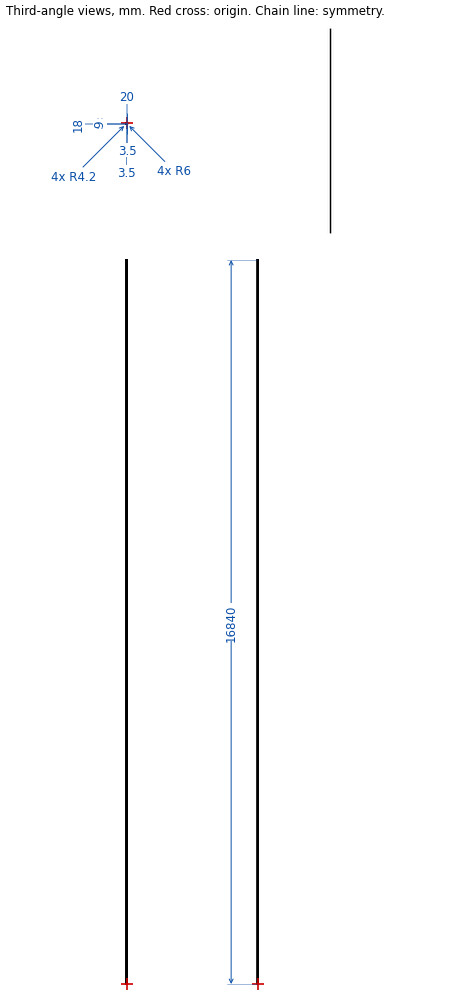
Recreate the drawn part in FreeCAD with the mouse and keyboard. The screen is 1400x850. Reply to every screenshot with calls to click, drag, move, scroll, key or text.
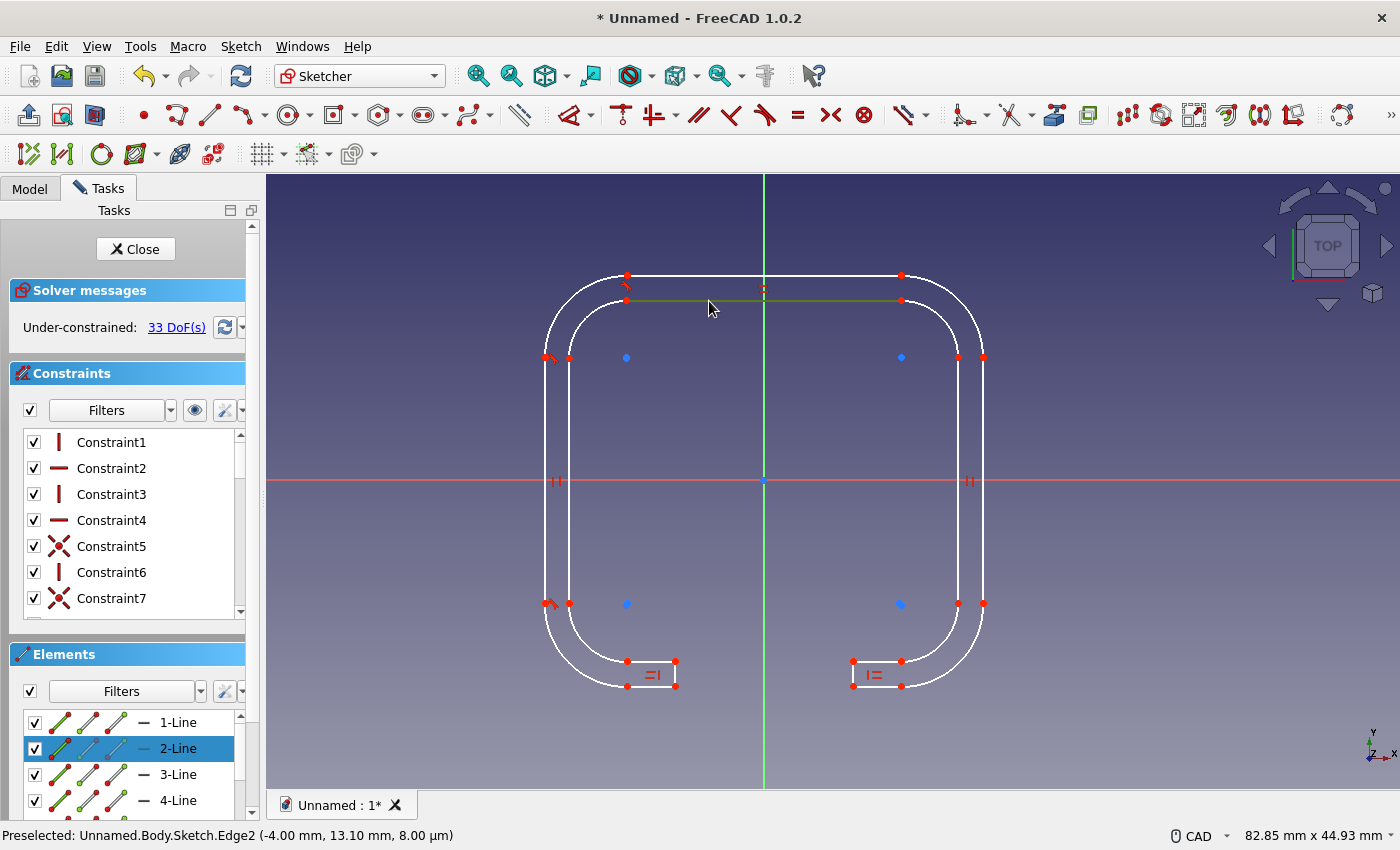
click(952, 332)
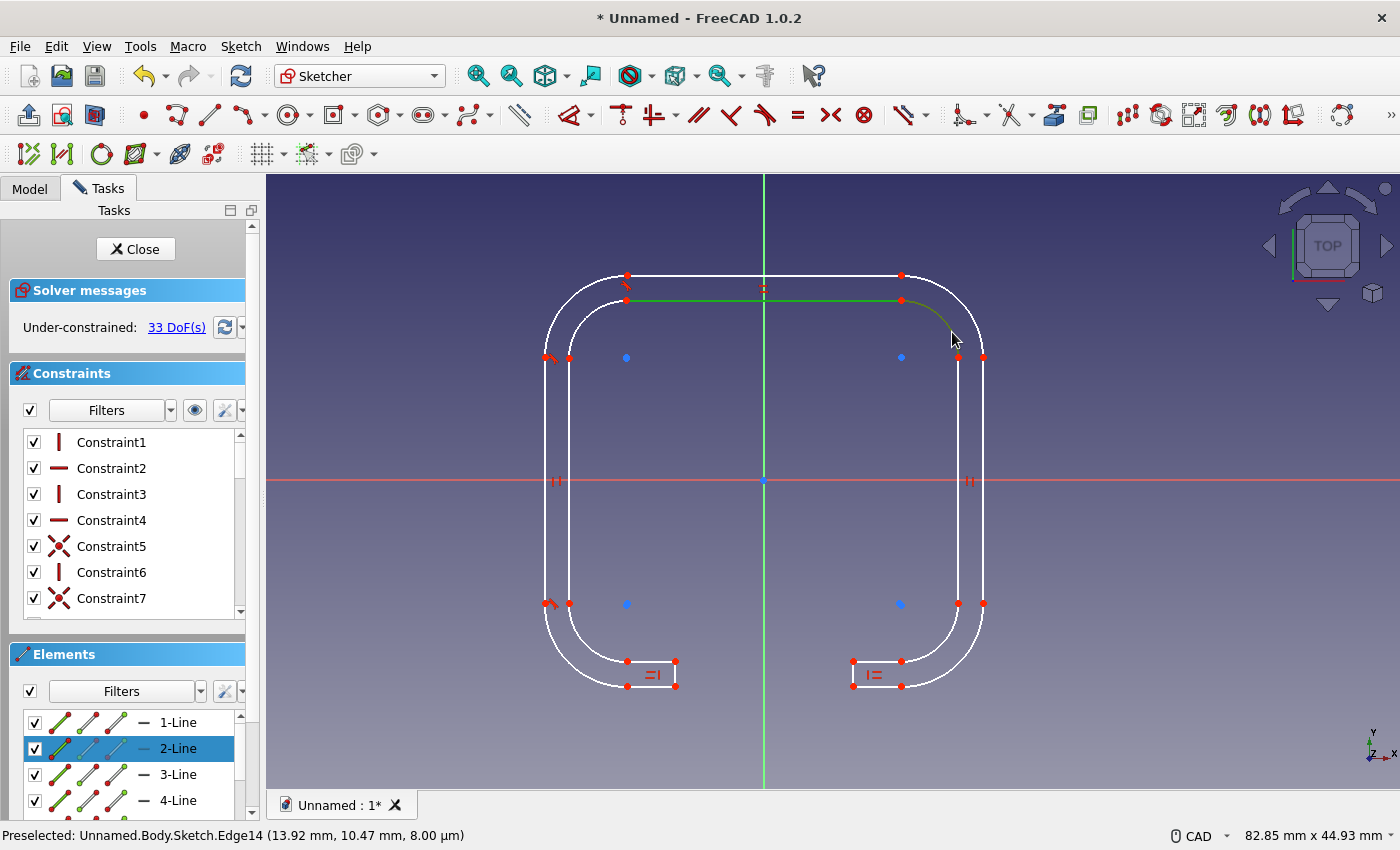
click(765, 116)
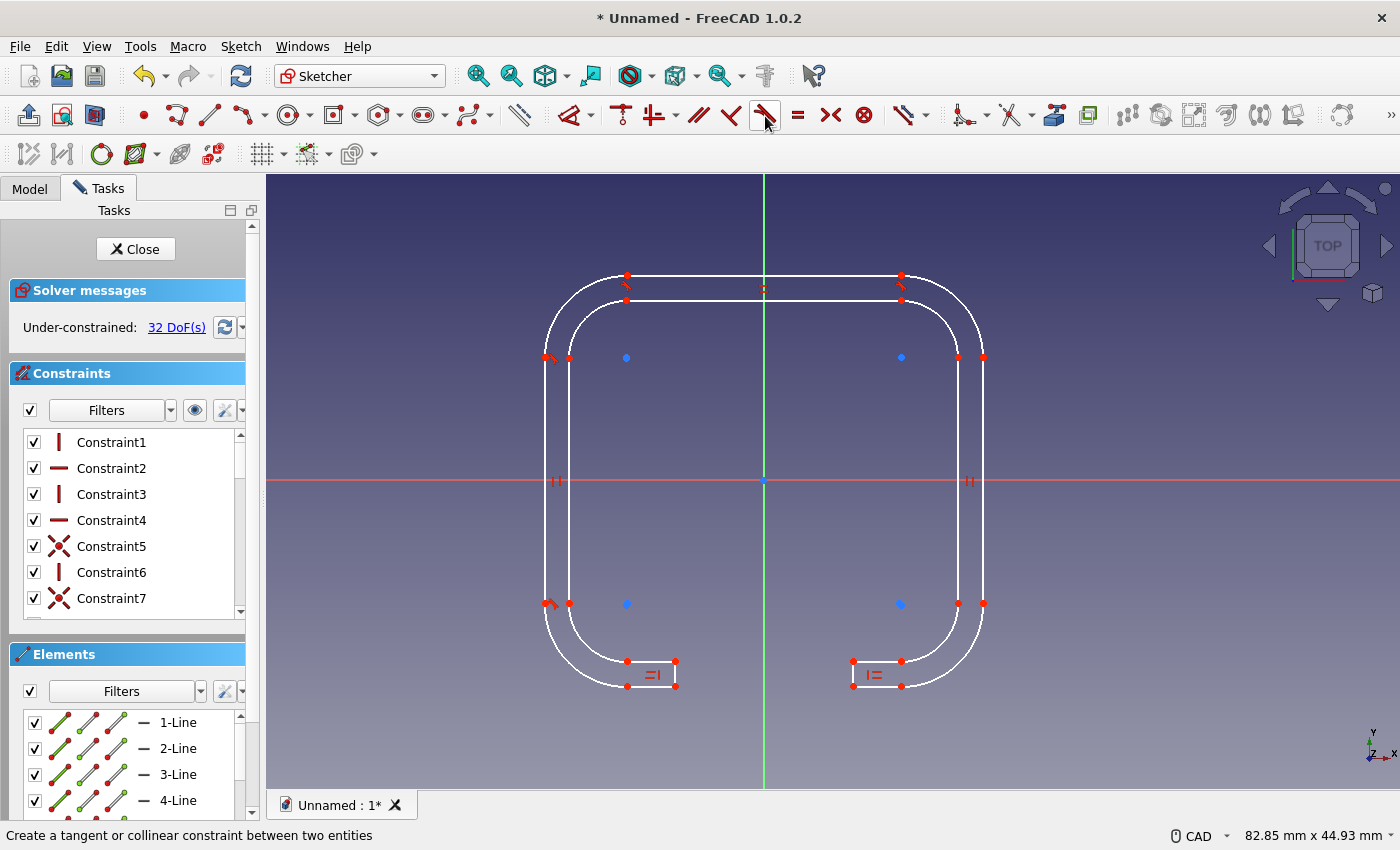
click(958, 432)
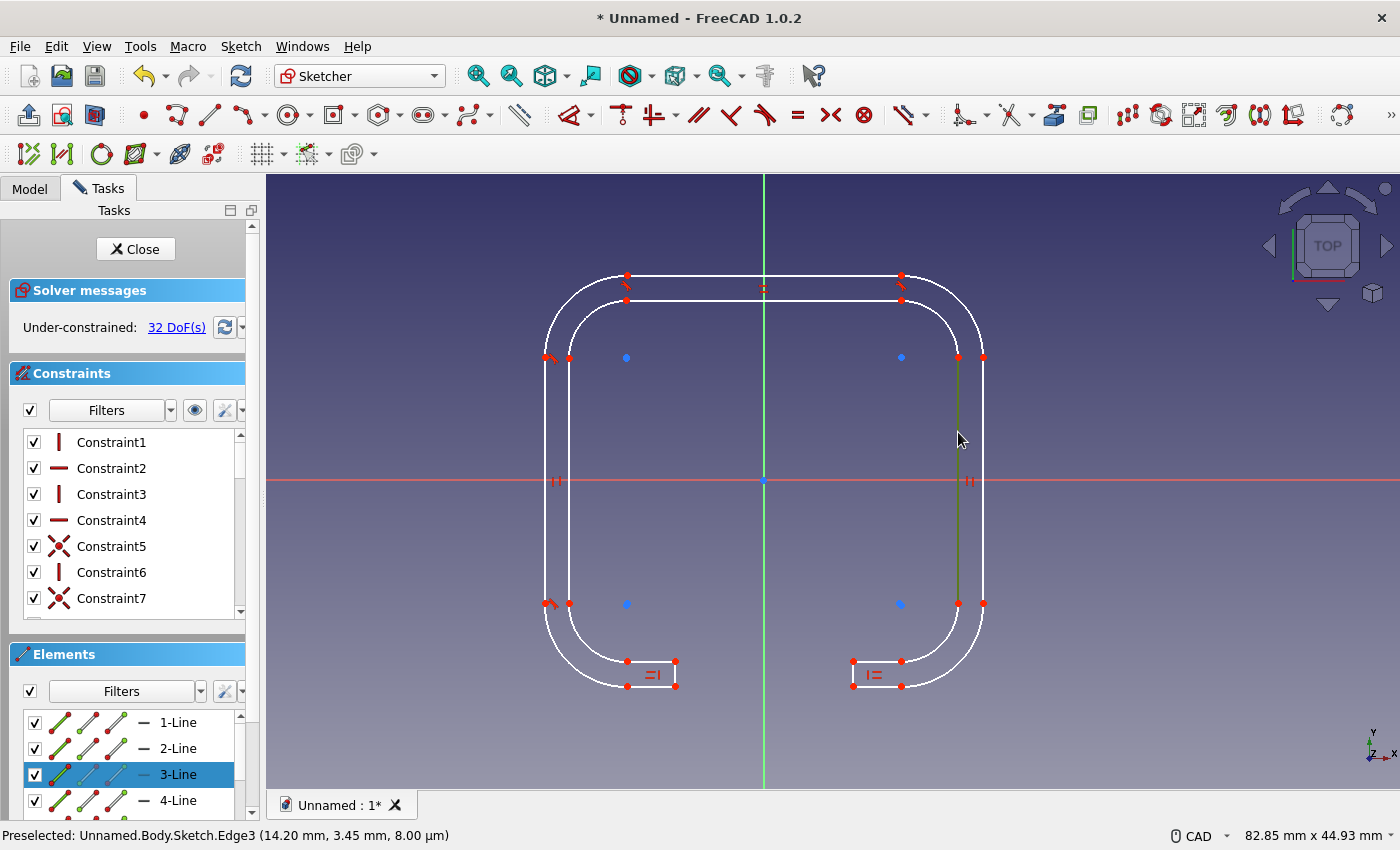
click(952, 332)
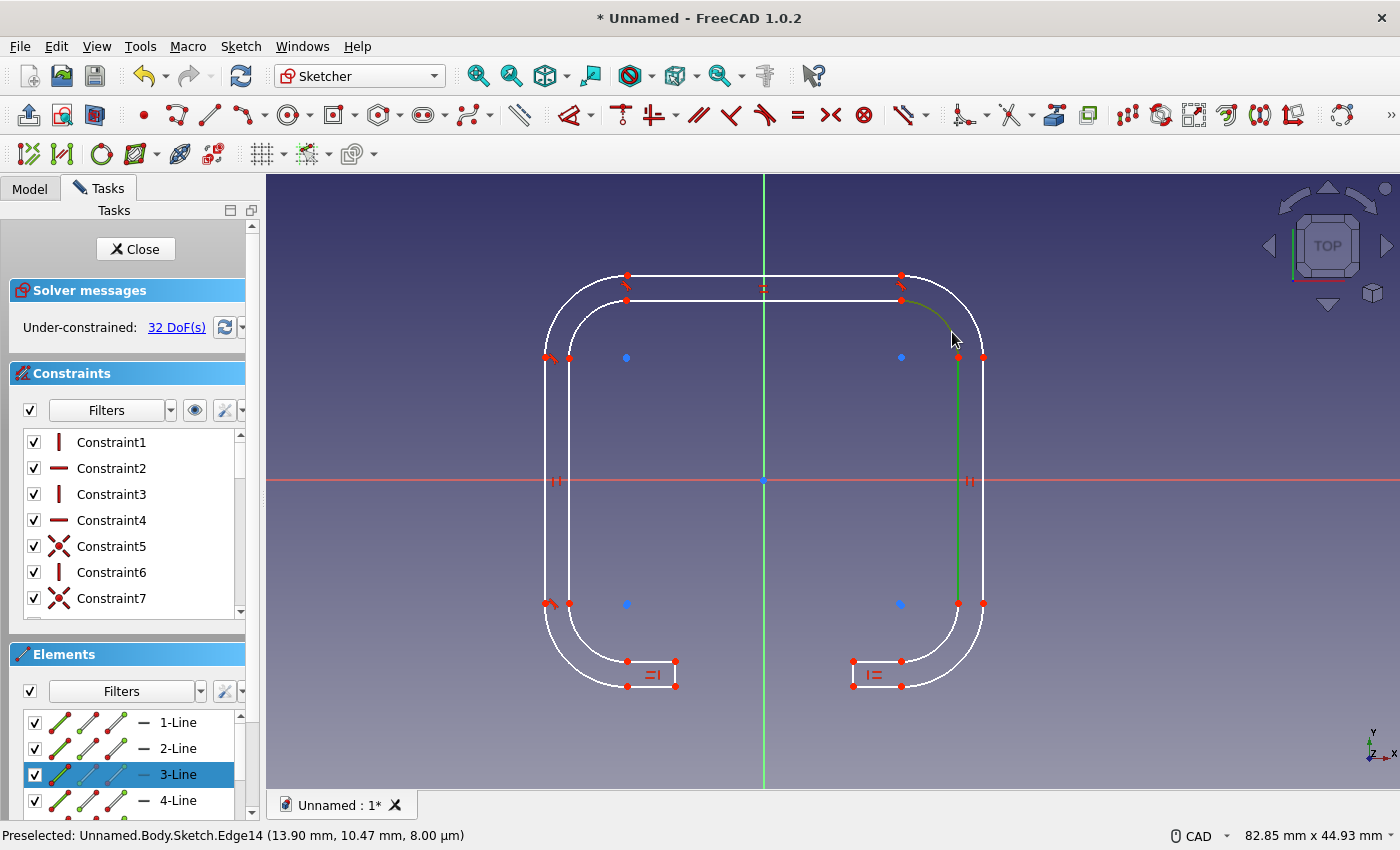
click(765, 116)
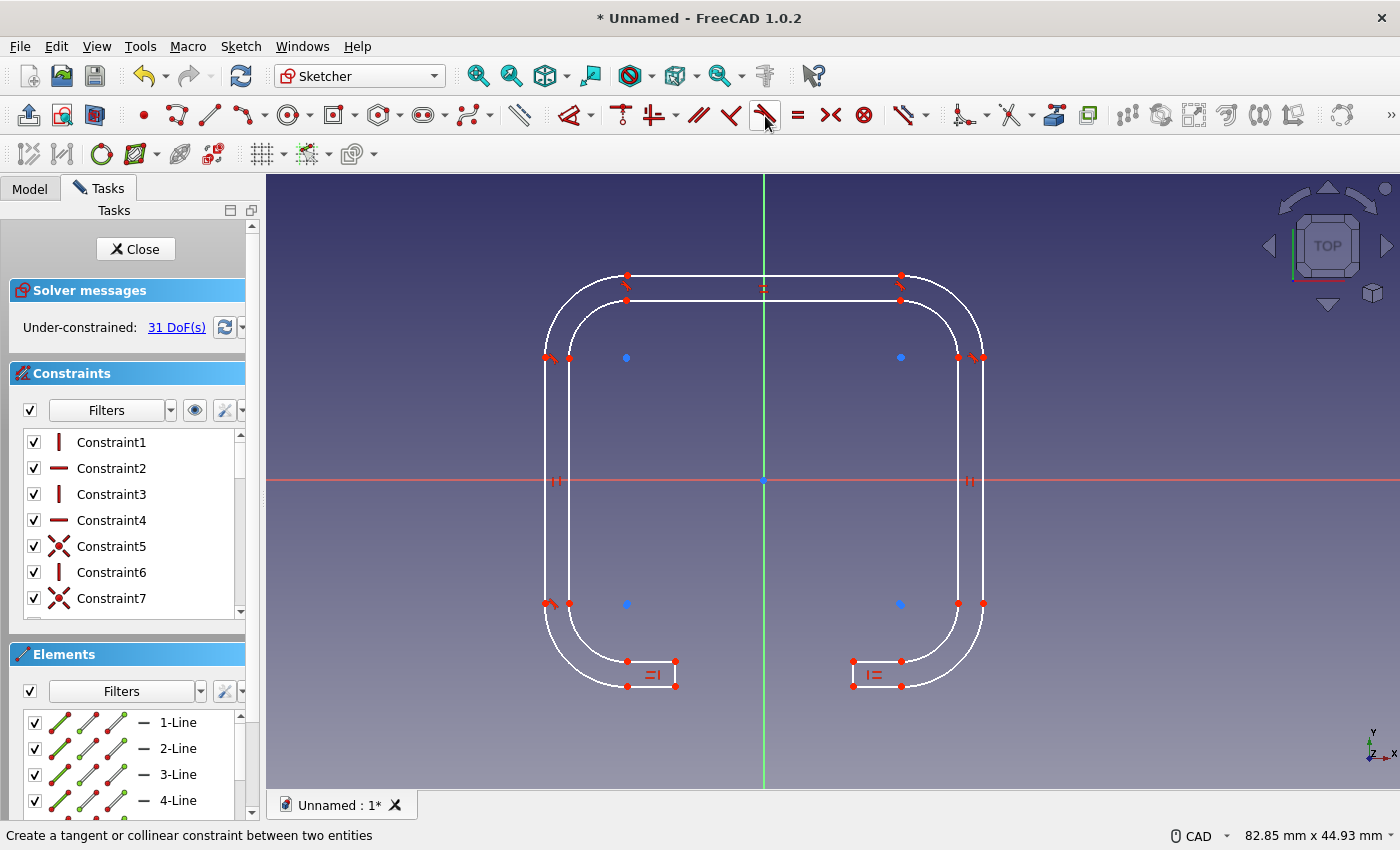
click(958, 432)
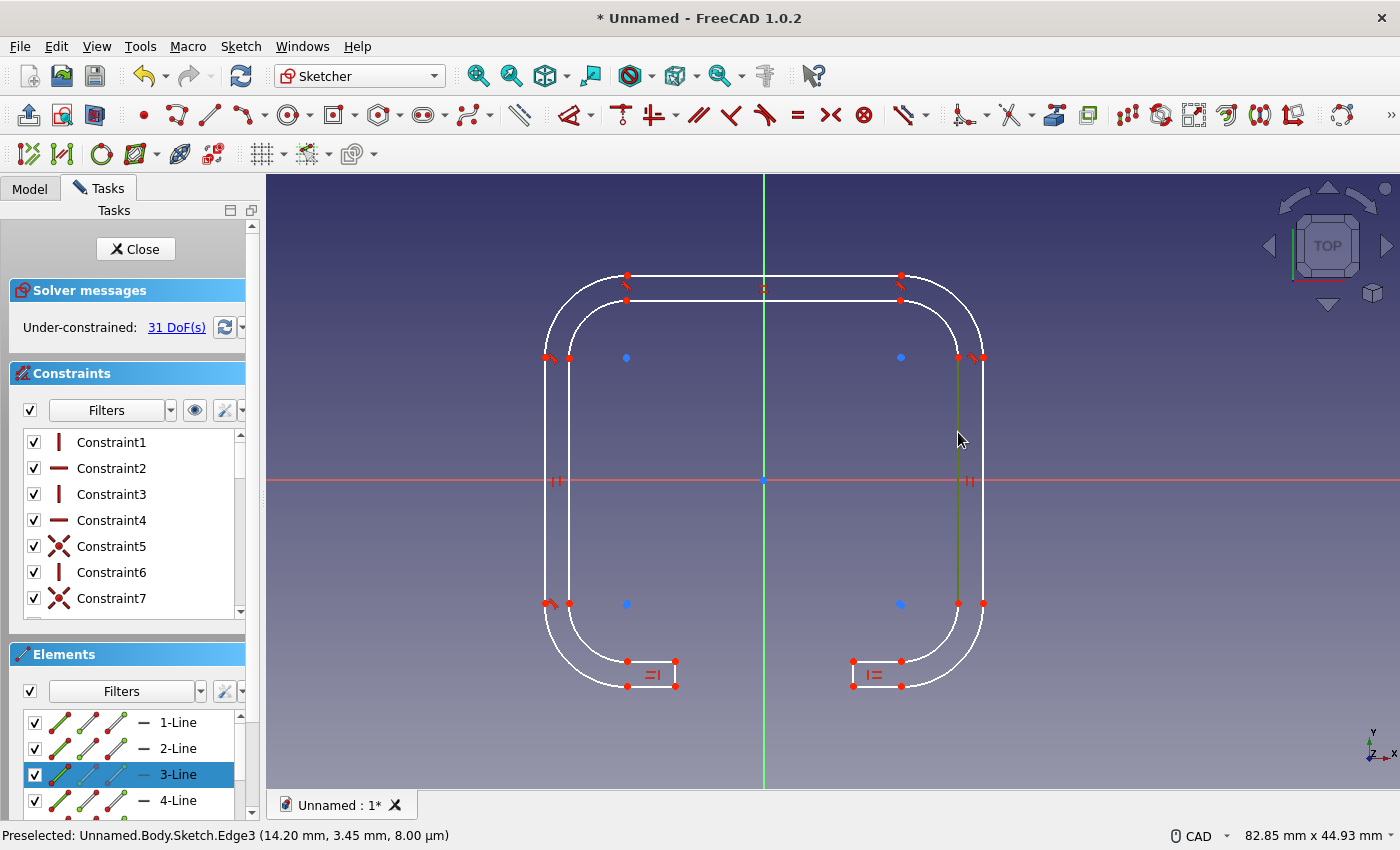
click(927, 655)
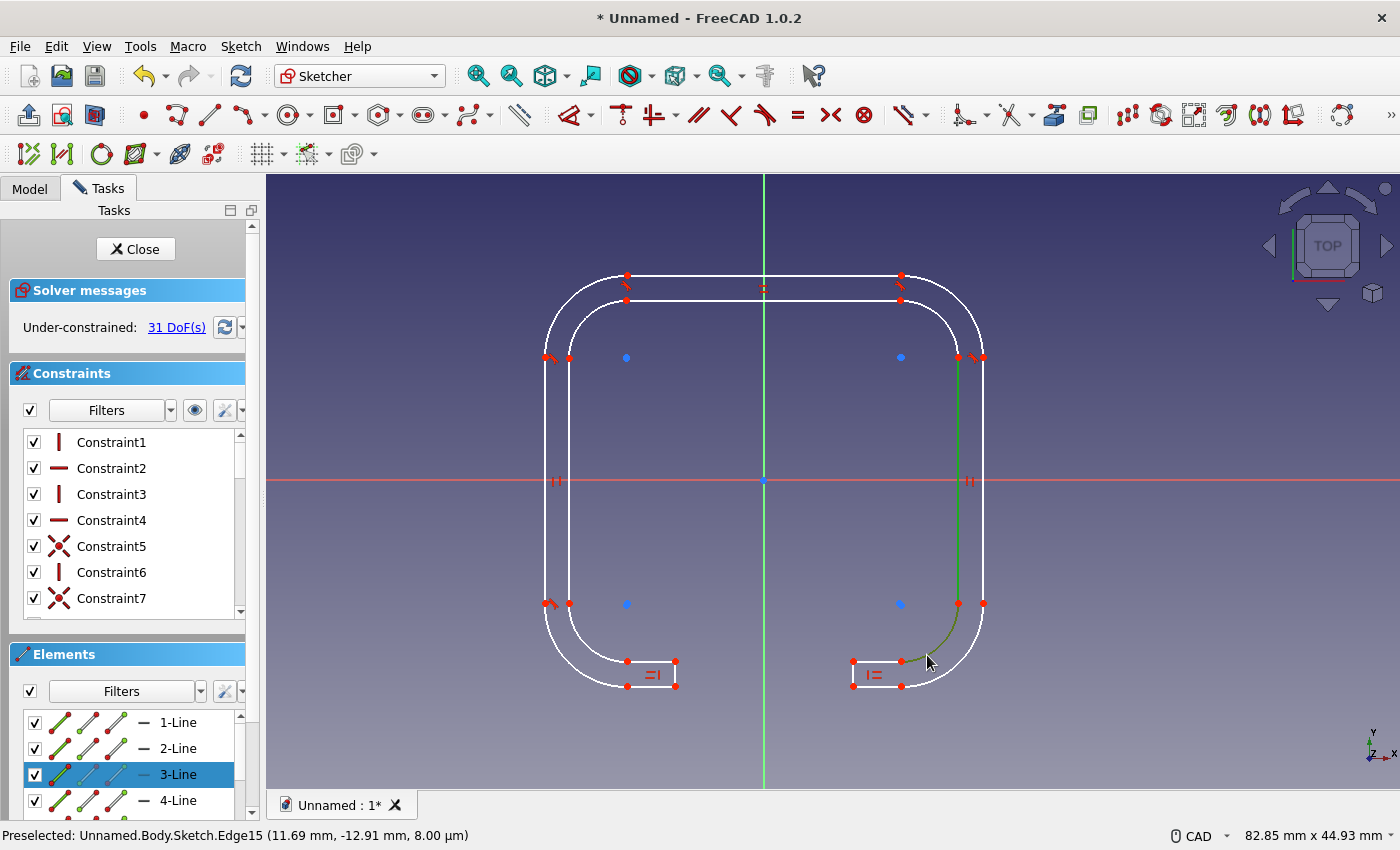
click(765, 116)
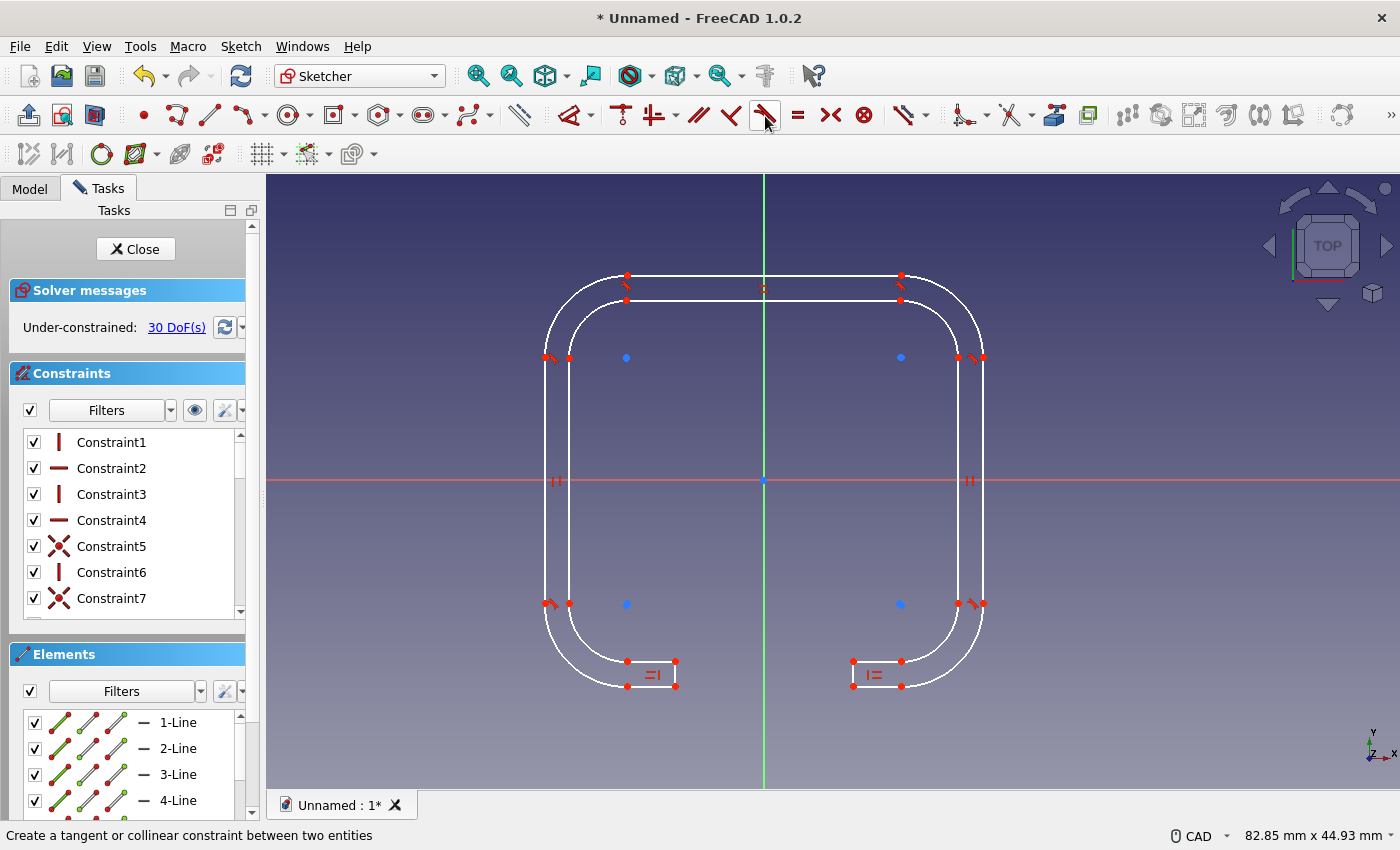
click(887, 662)